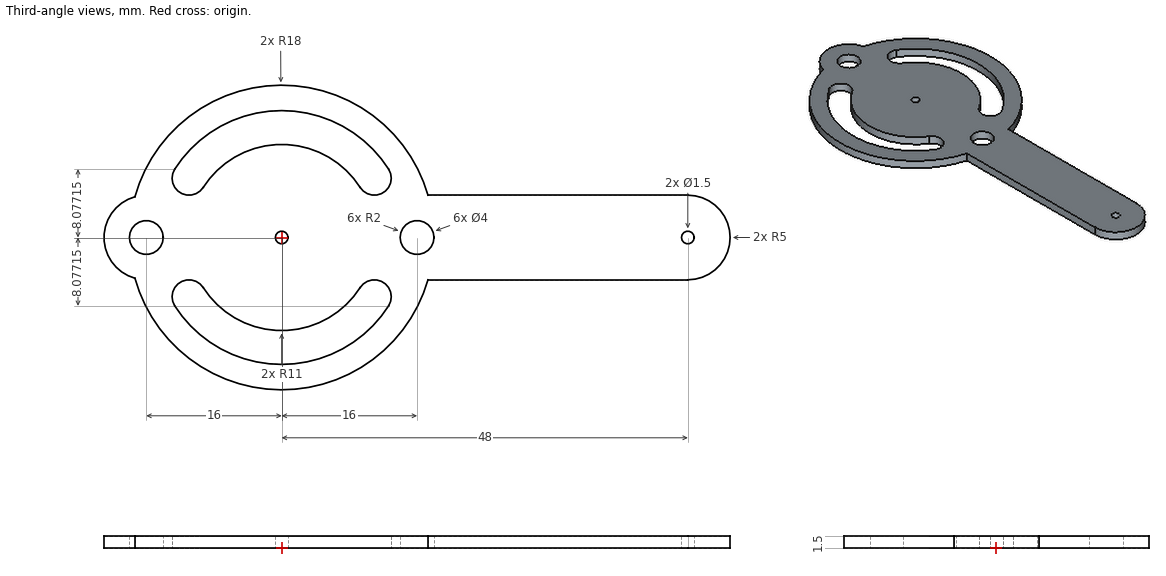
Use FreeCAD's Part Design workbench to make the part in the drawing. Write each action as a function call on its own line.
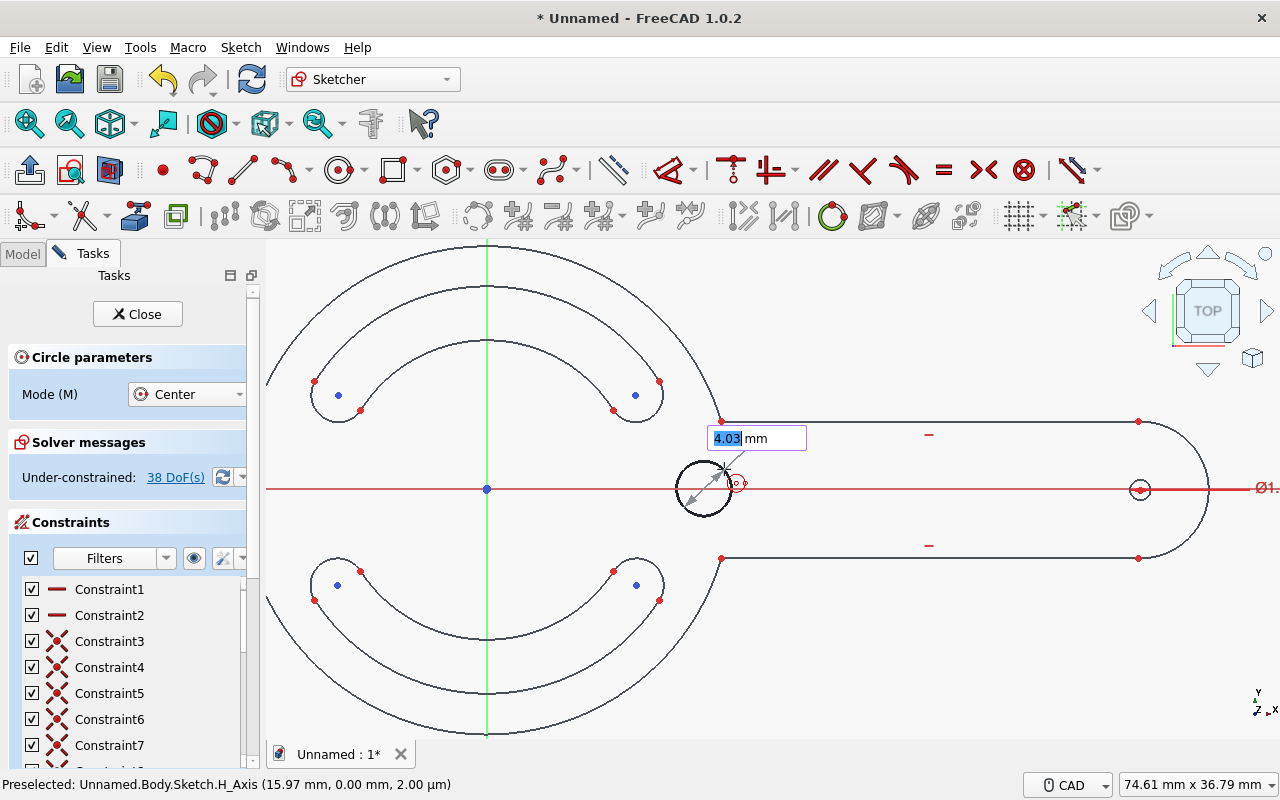
text(4)
key(Return)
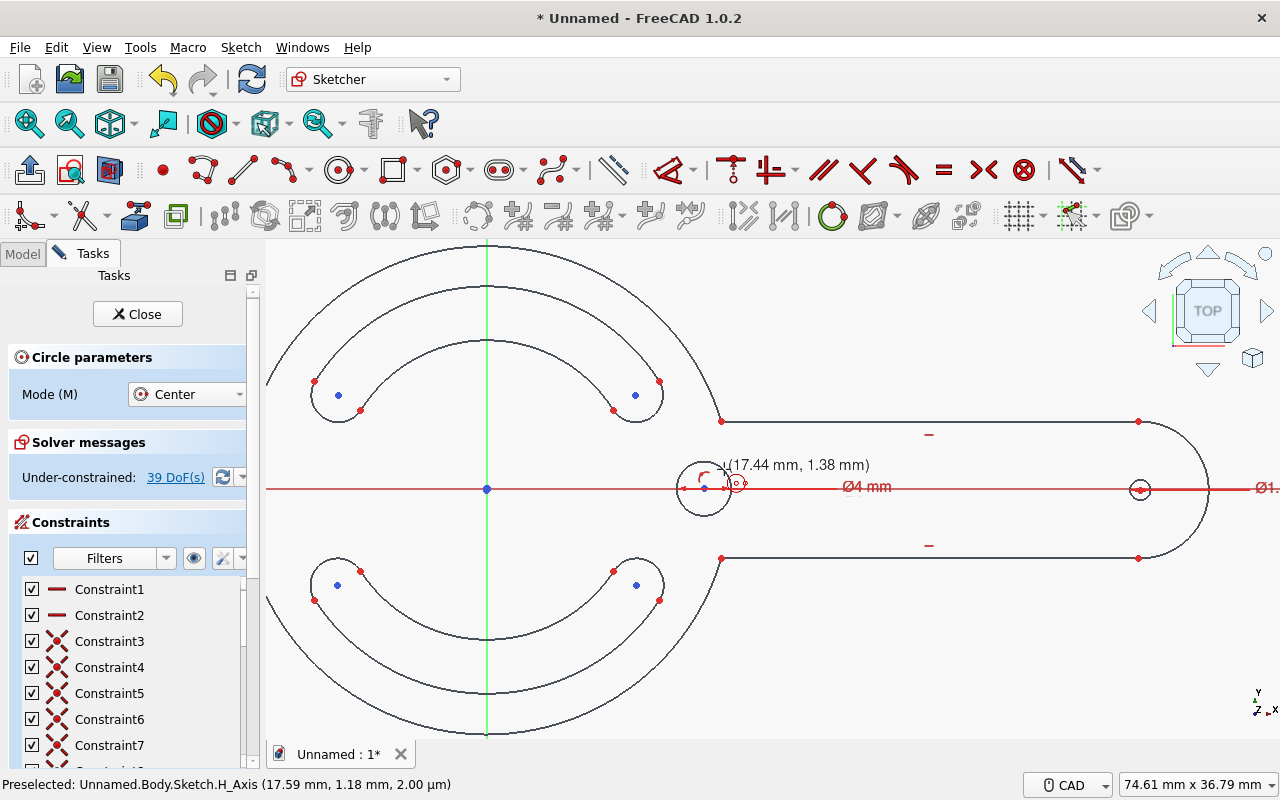
scroll(487, 489, up, 4)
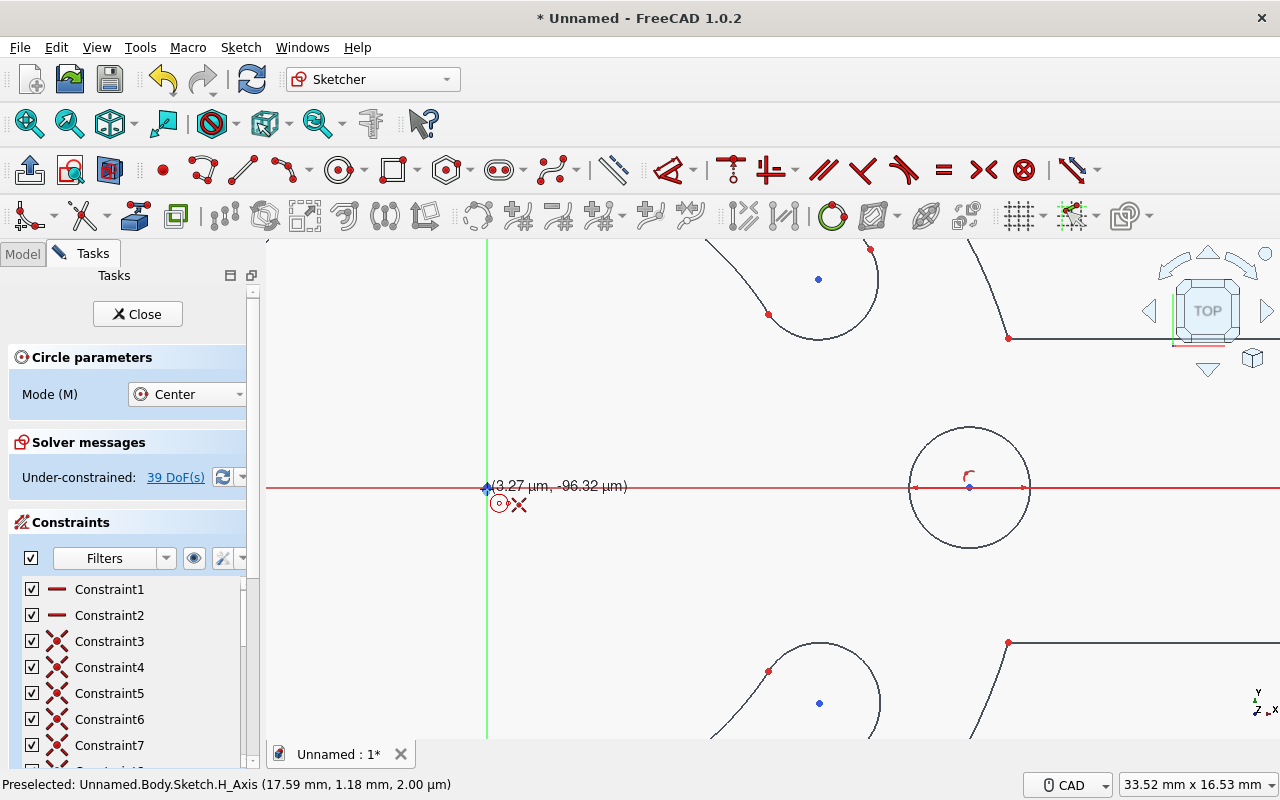
scroll(617, 489, down, 7)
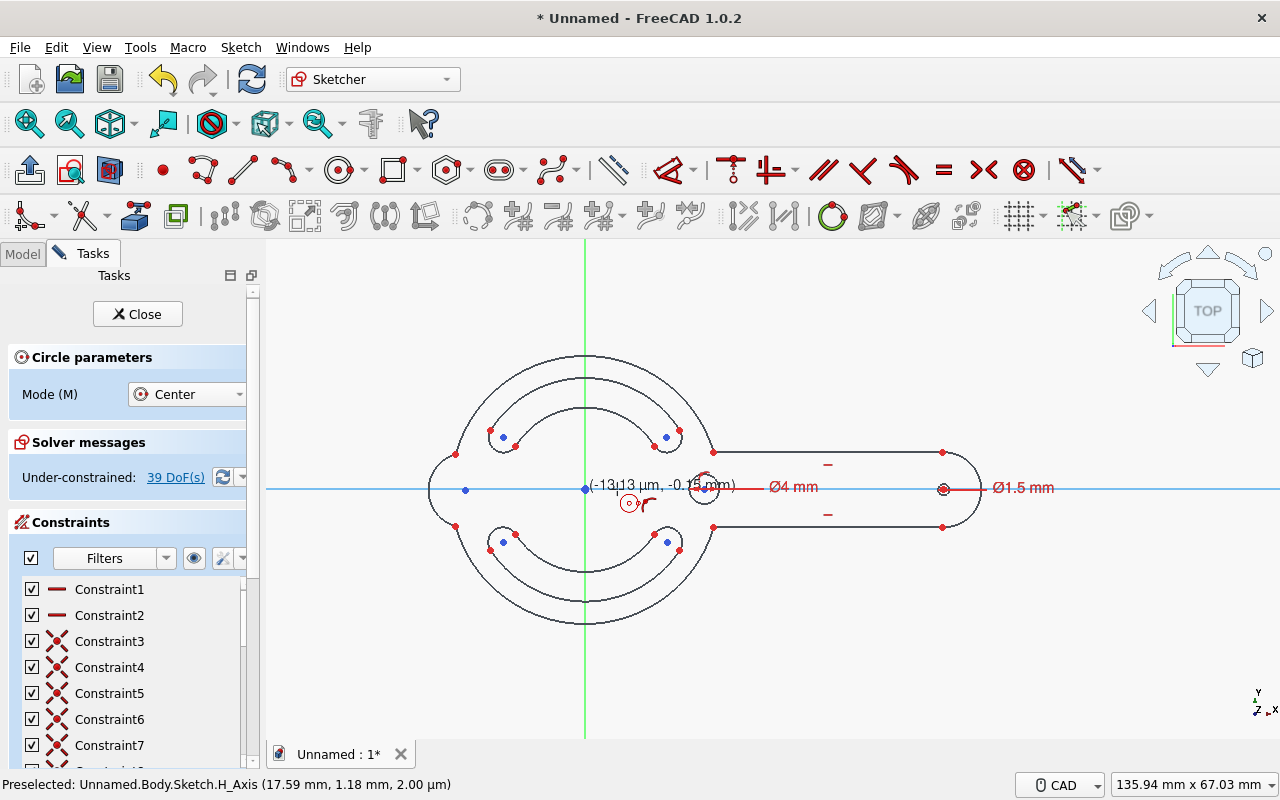
click(585, 489)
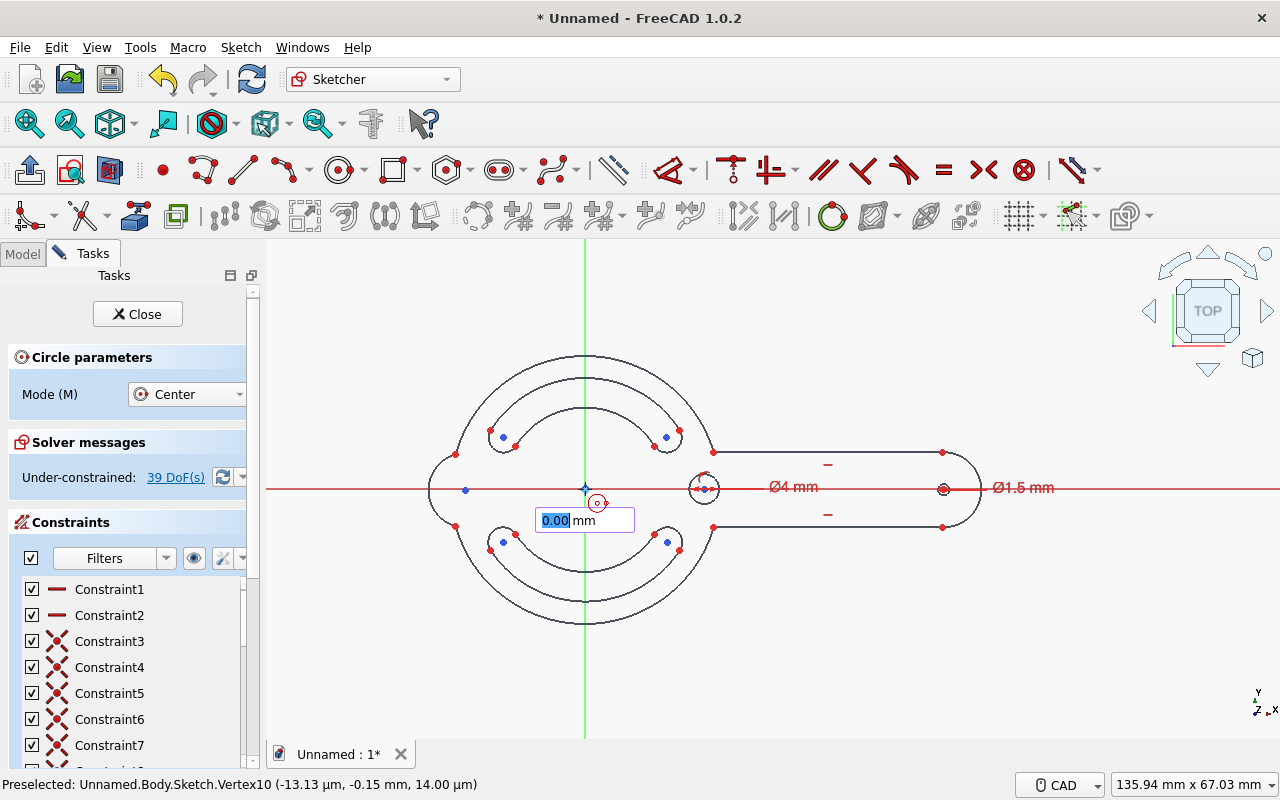
scroll(589, 485, up, 7)
move(588, 484)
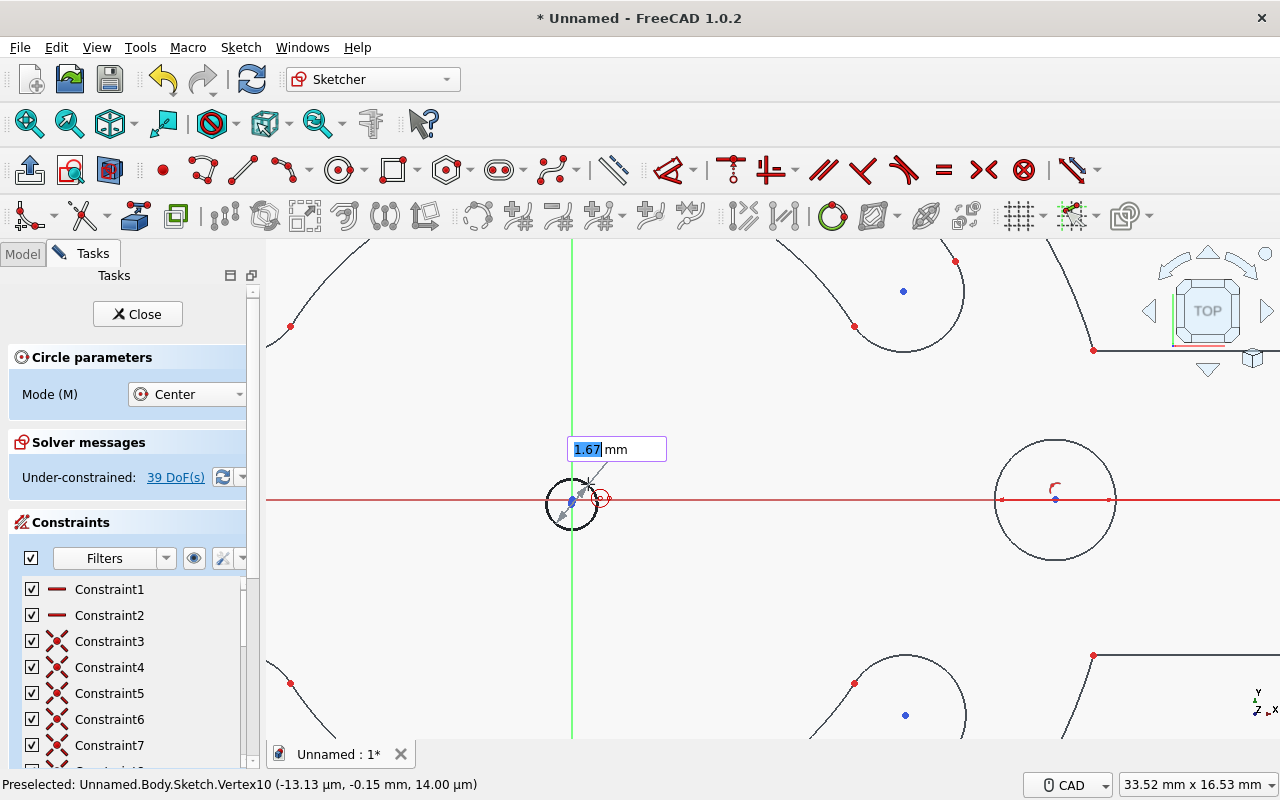
text(1.5)
key(Return)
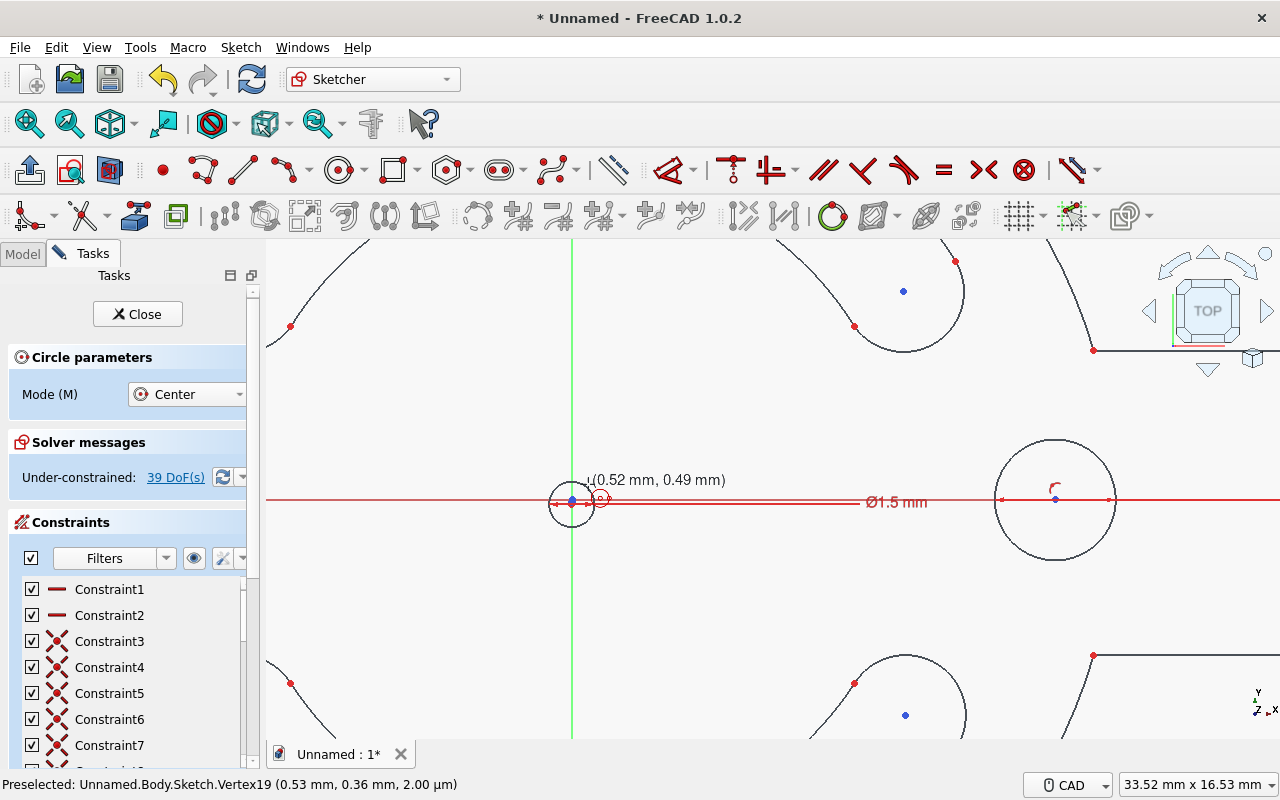
scroll(589, 485, down, 7)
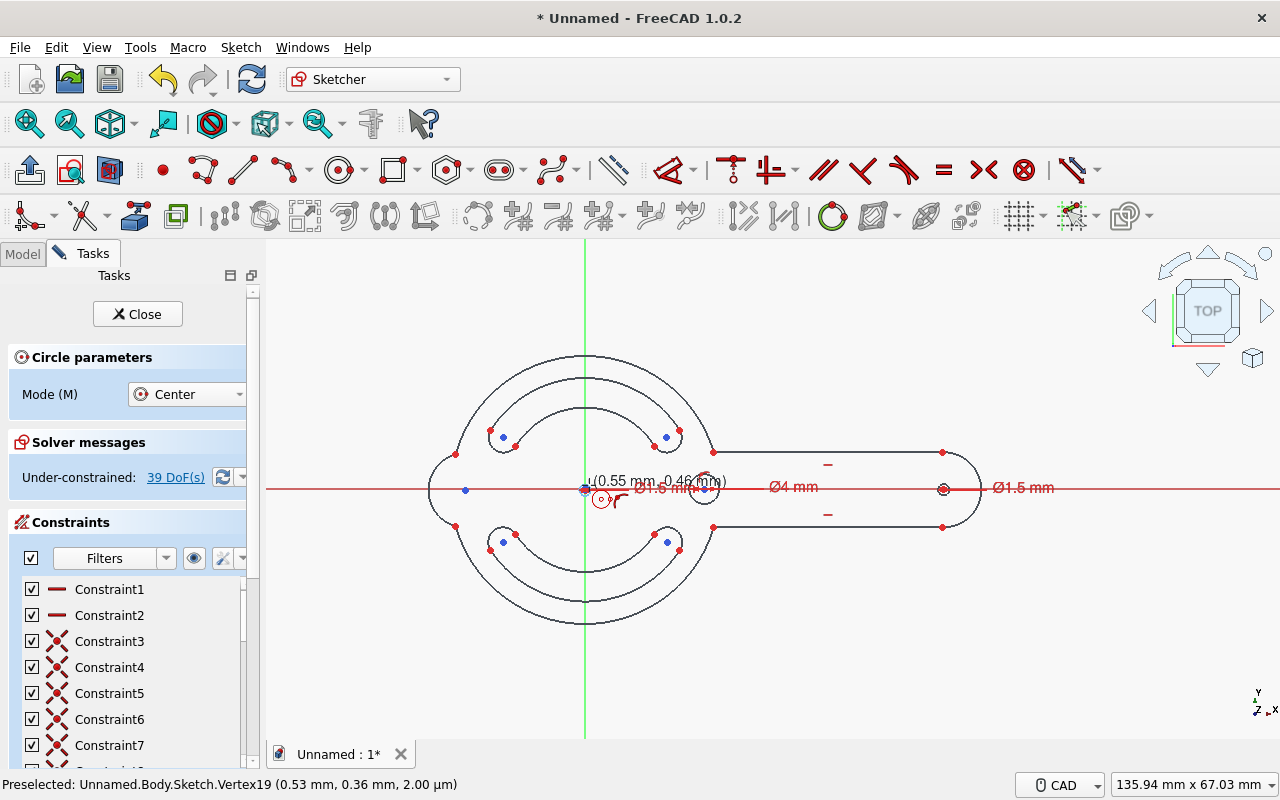
scroll(466, 489, up, 3)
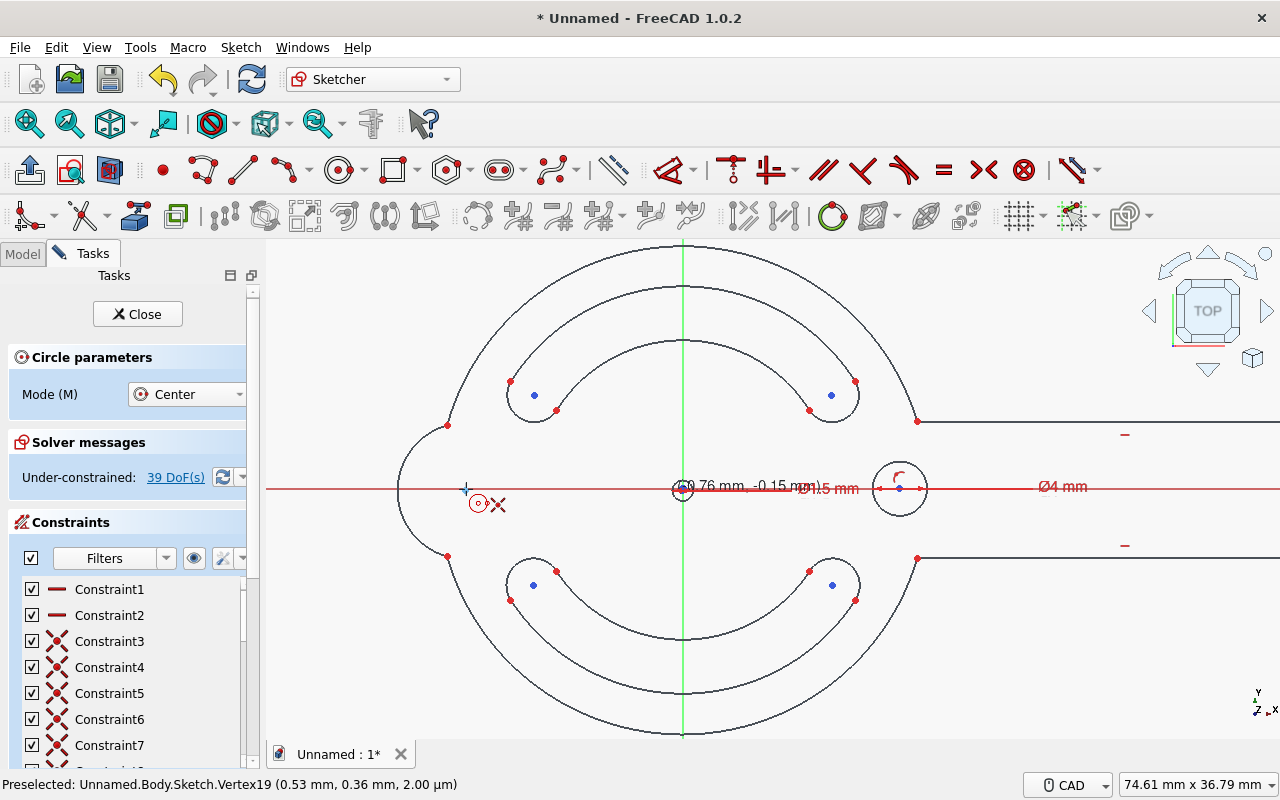
click(465, 489)
move(485, 469)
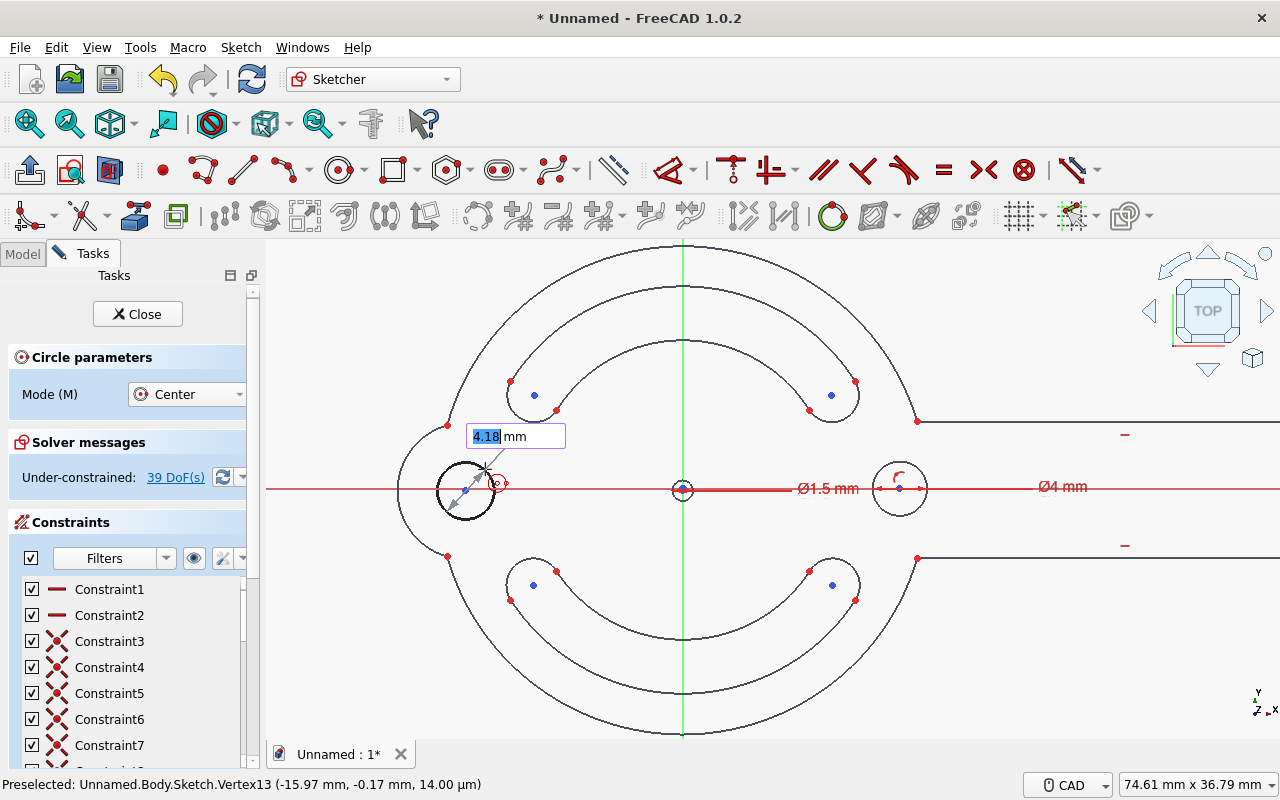
text(4)
key(Return)
key(Escape)